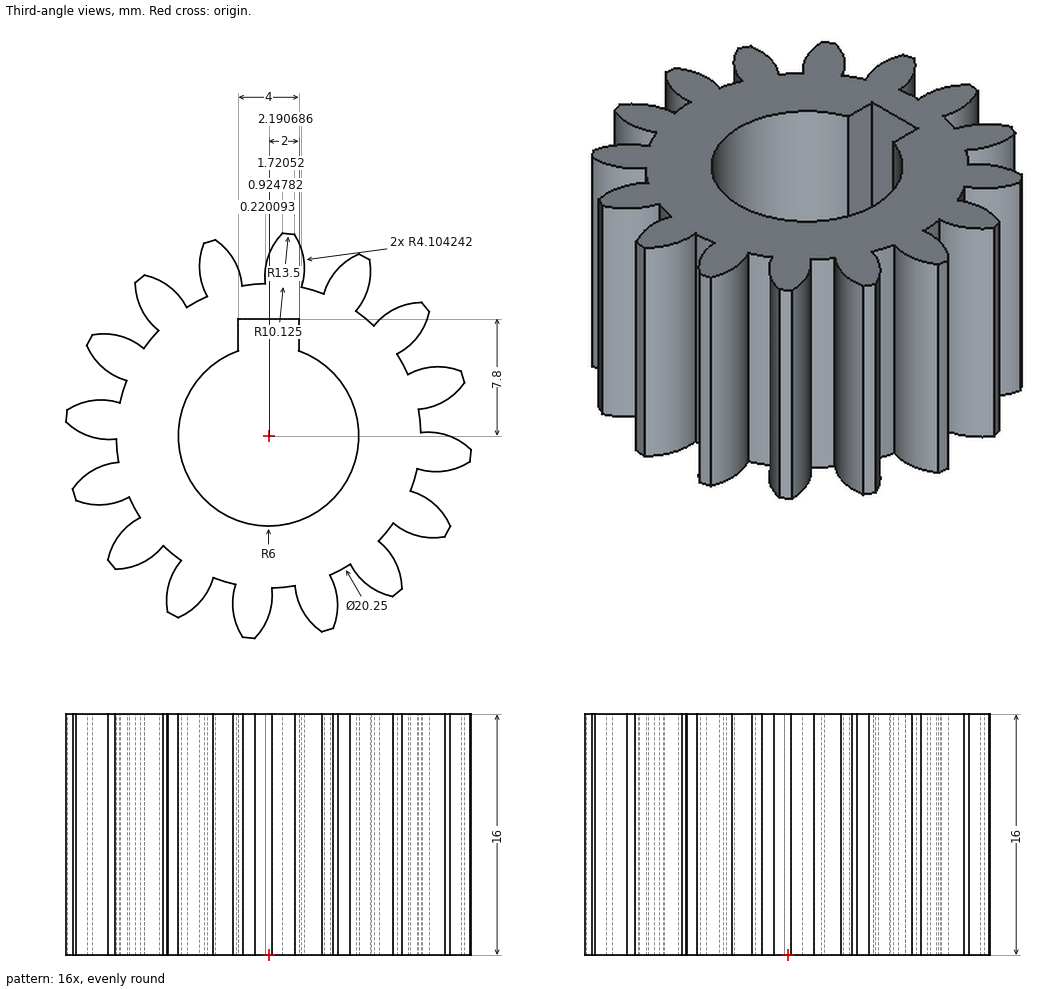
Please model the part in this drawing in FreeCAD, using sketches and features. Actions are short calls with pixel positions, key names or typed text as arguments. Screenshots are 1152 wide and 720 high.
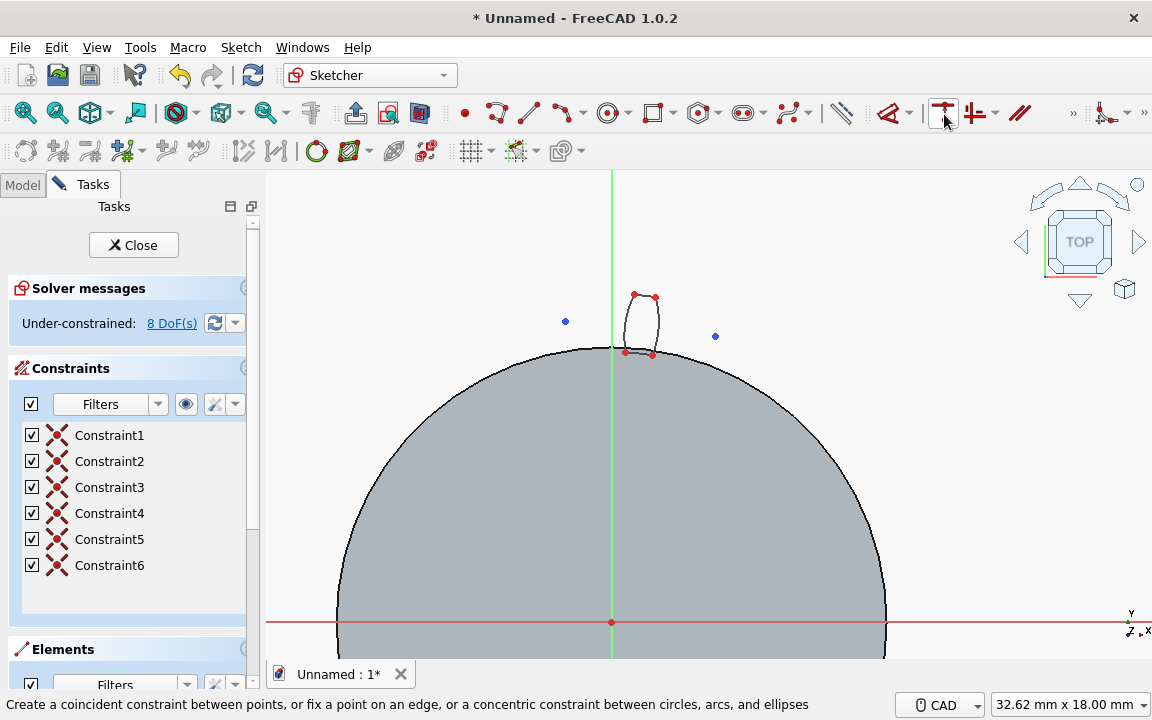
click(657, 338)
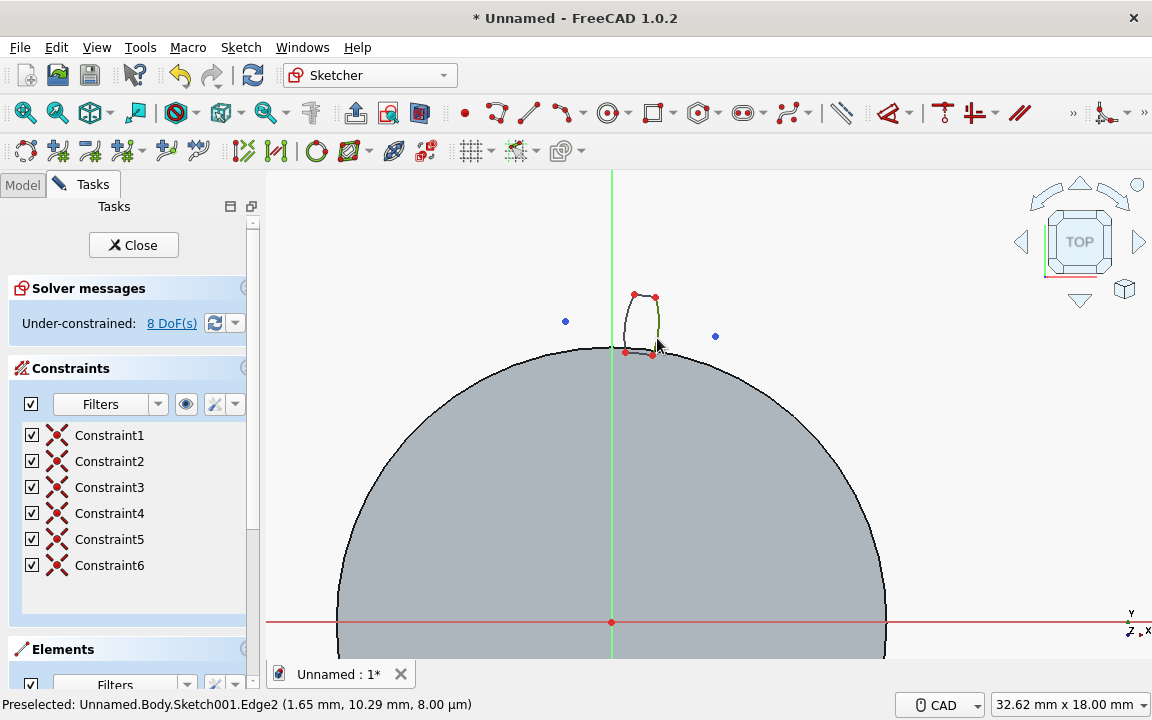
click(628, 311)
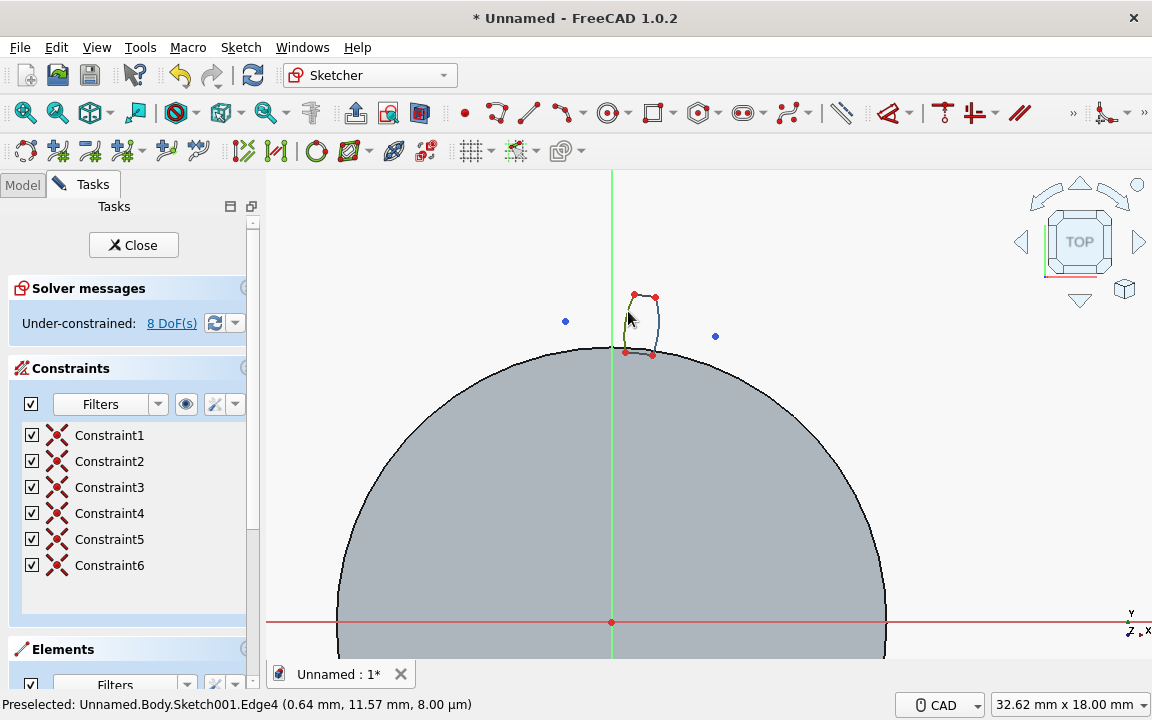
key(e)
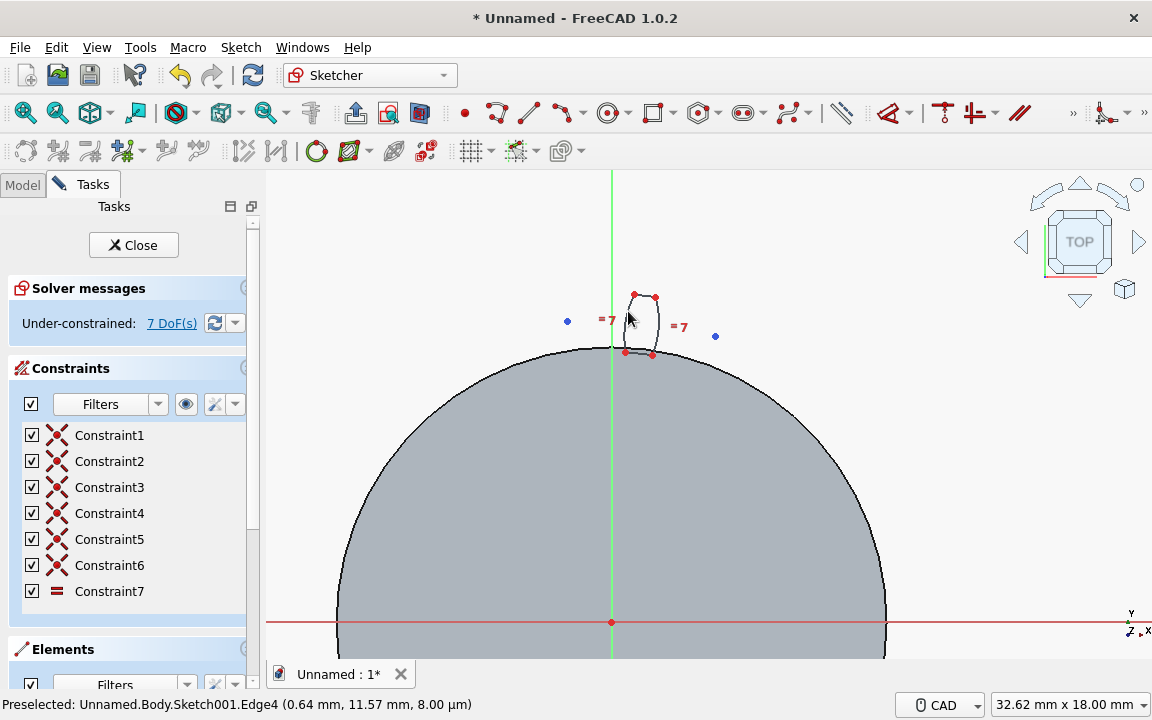
click(888, 114)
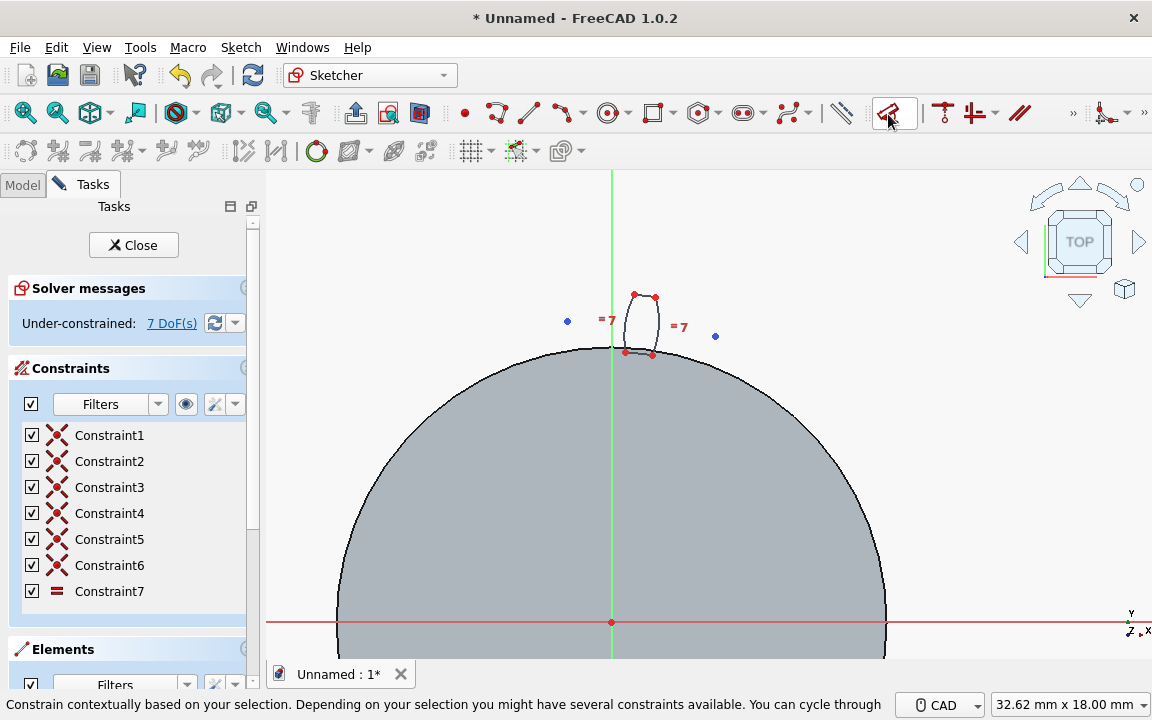
click(639, 354)
click(642, 322)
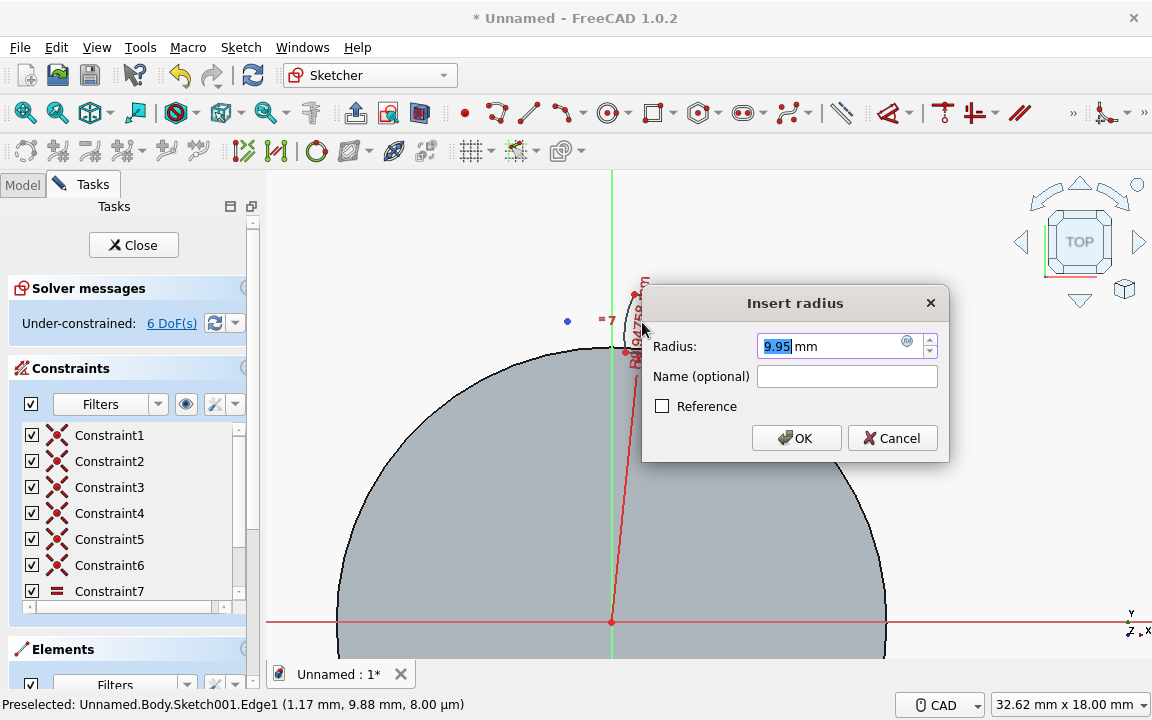
text(10.125)
key(Return)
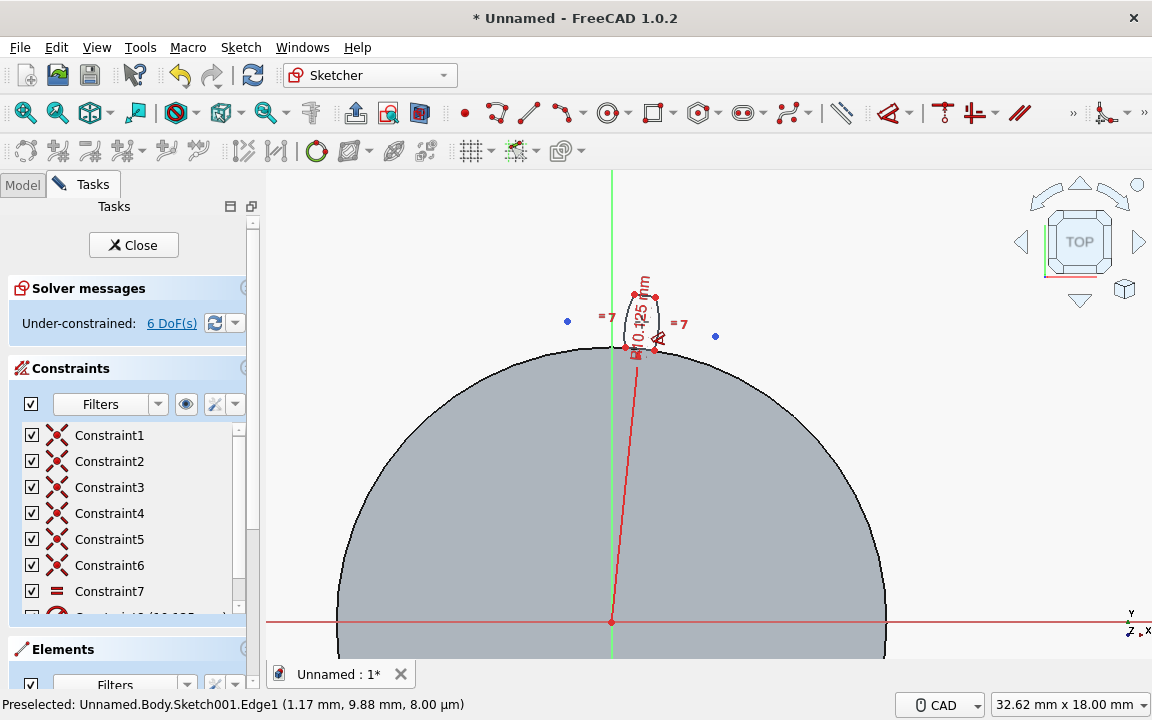
click(658, 335)
click(666, 396)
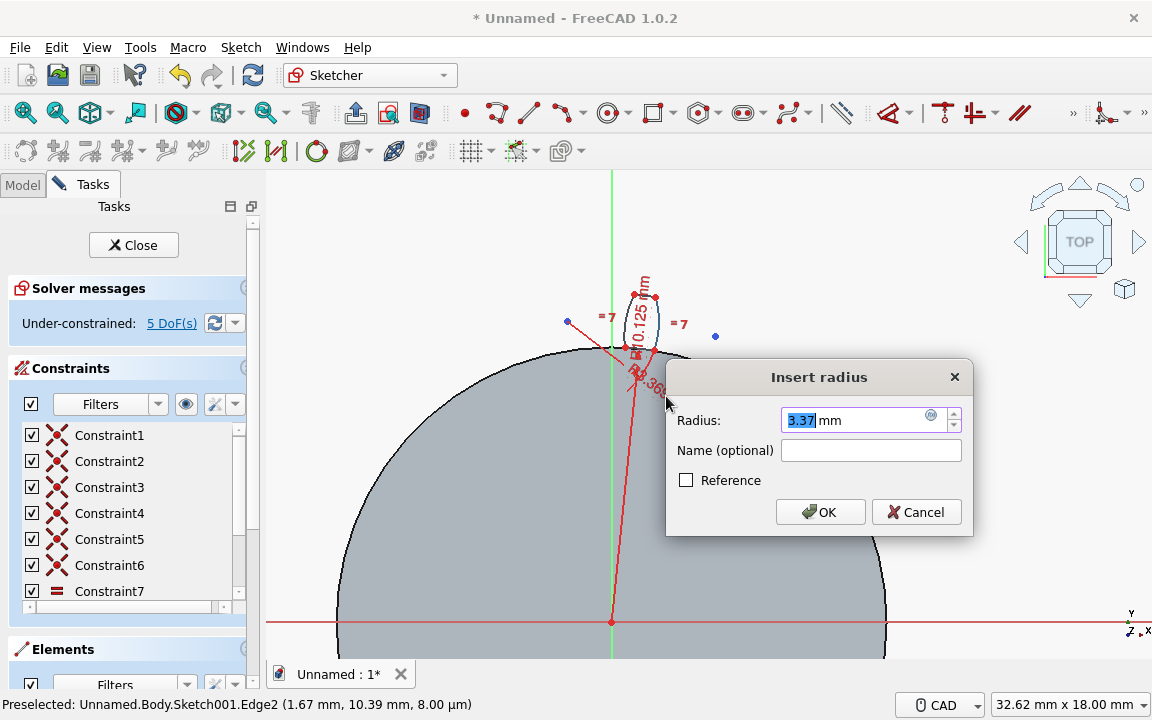
text(4.104242)
key(Return)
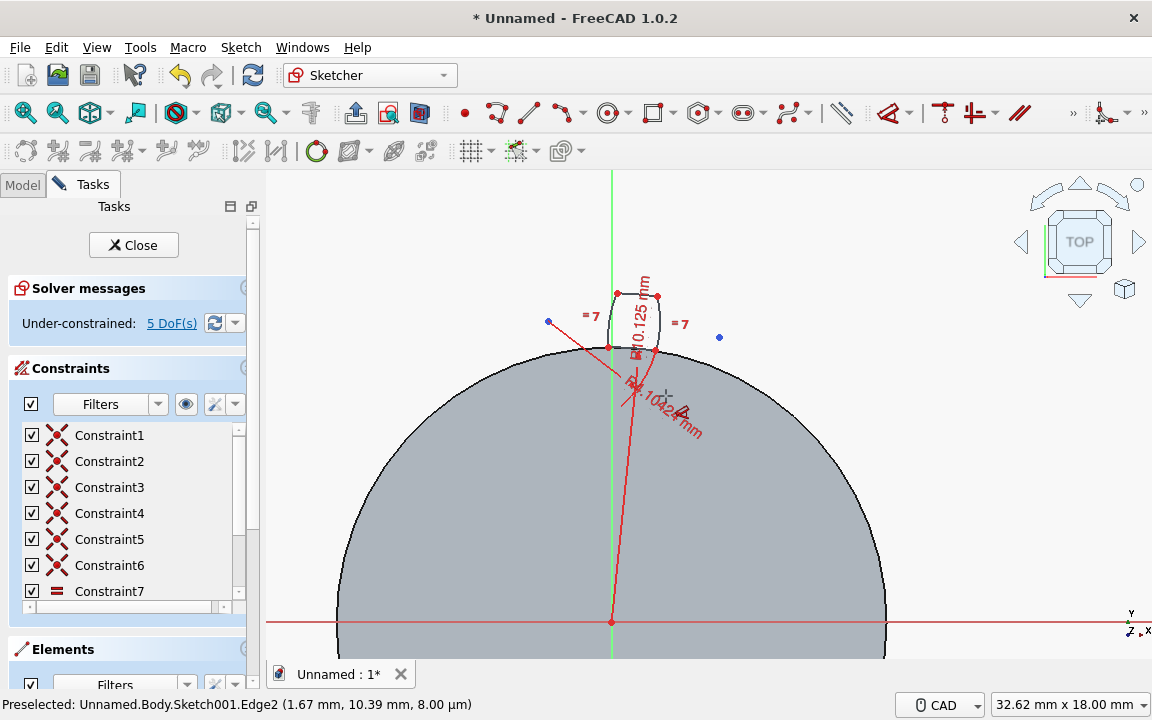
click(645, 295)
click(648, 263)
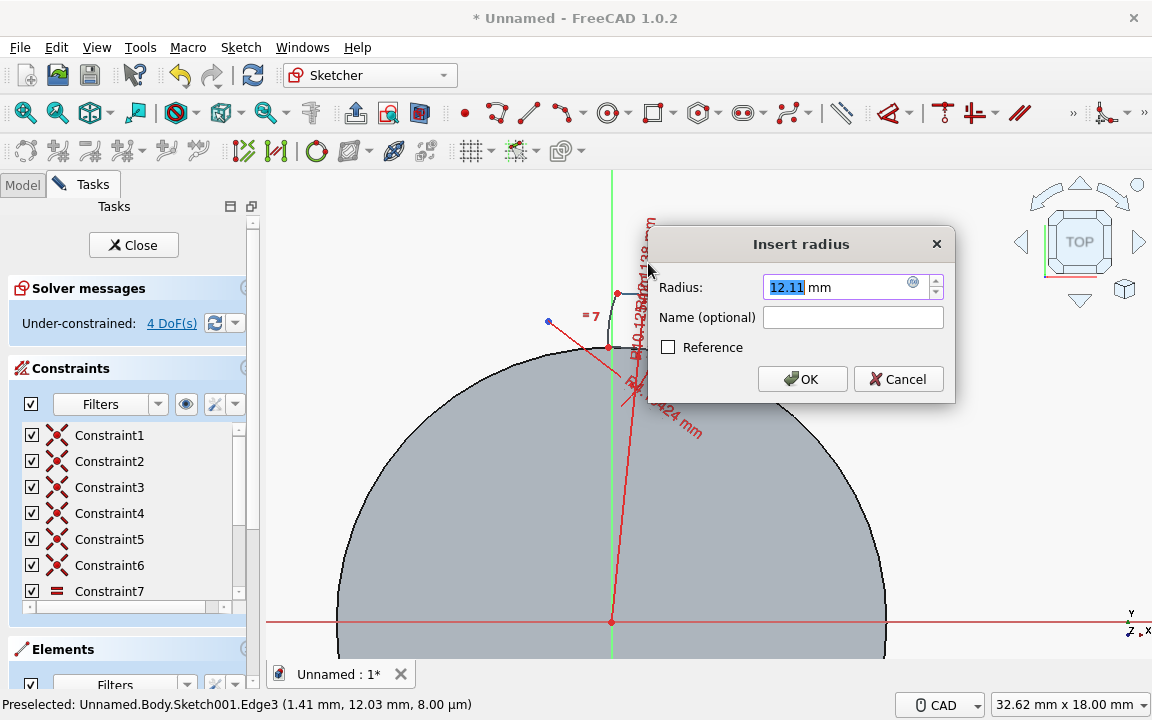
text(13.5)
key(Return)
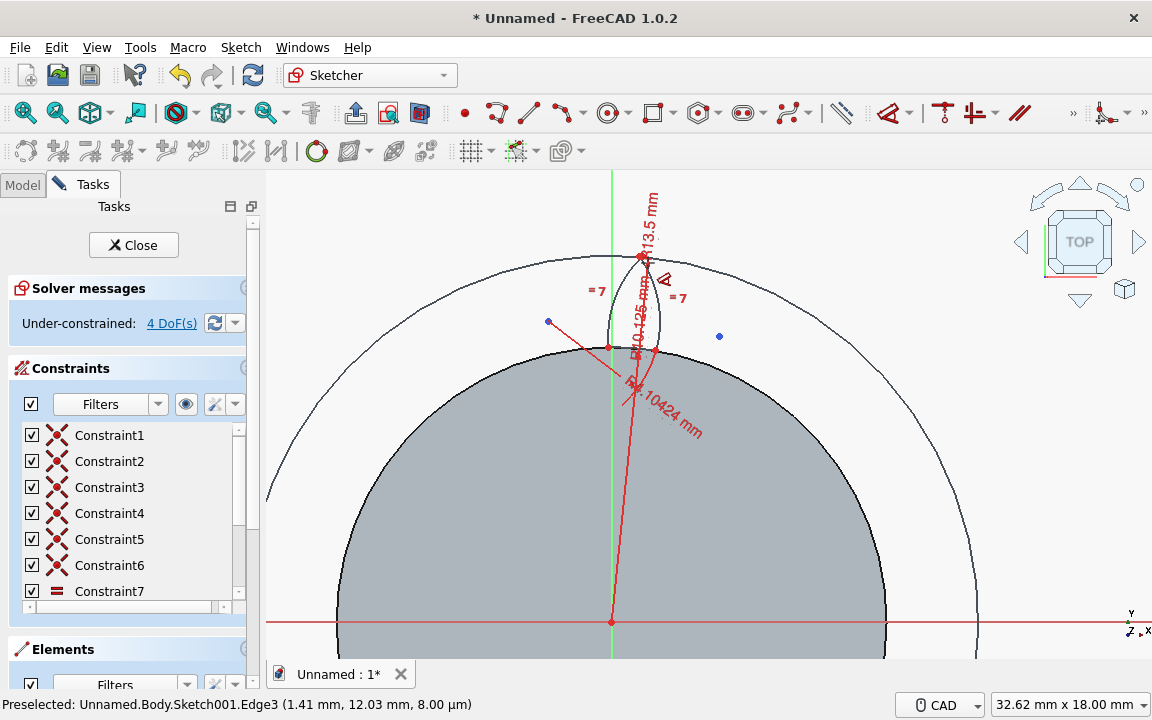
scroll(639, 257, up, 8)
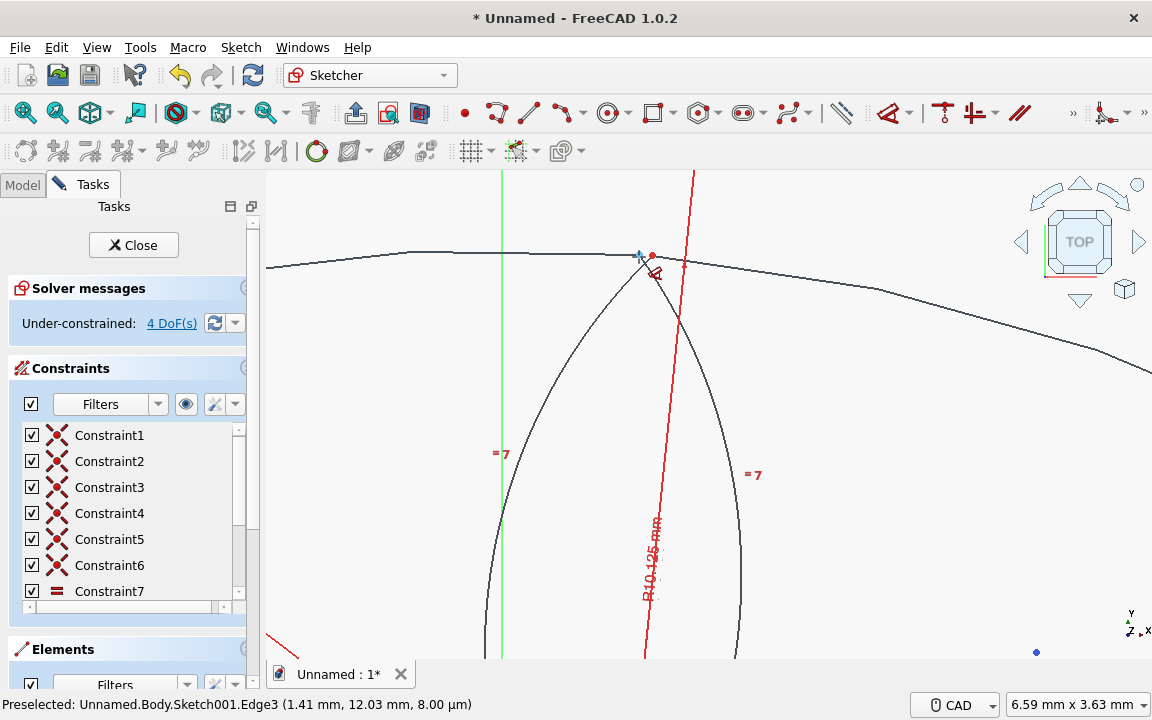
click(639, 255)
click(570, 221)